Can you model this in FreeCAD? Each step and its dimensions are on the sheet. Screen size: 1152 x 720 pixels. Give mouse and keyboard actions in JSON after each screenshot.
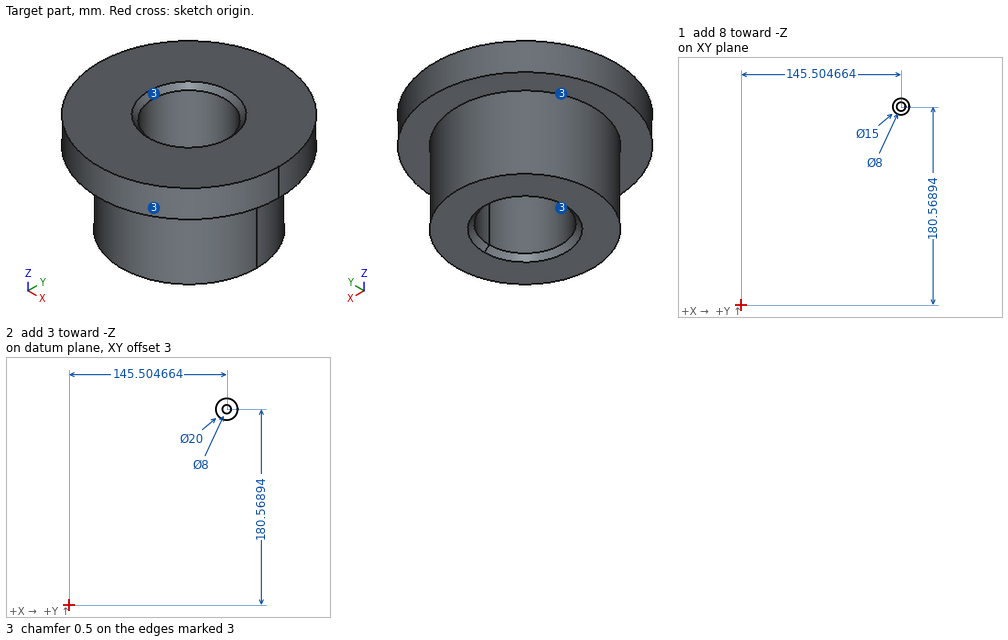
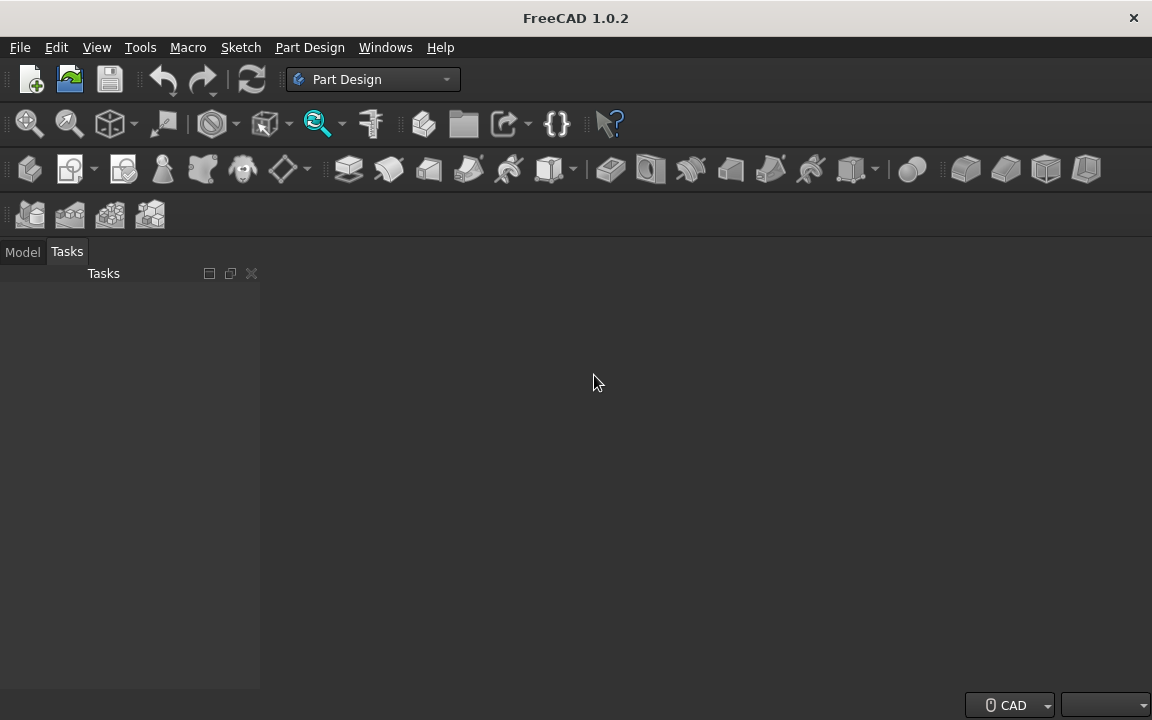
{"action": "left_click", "coordinate": [30, 80]}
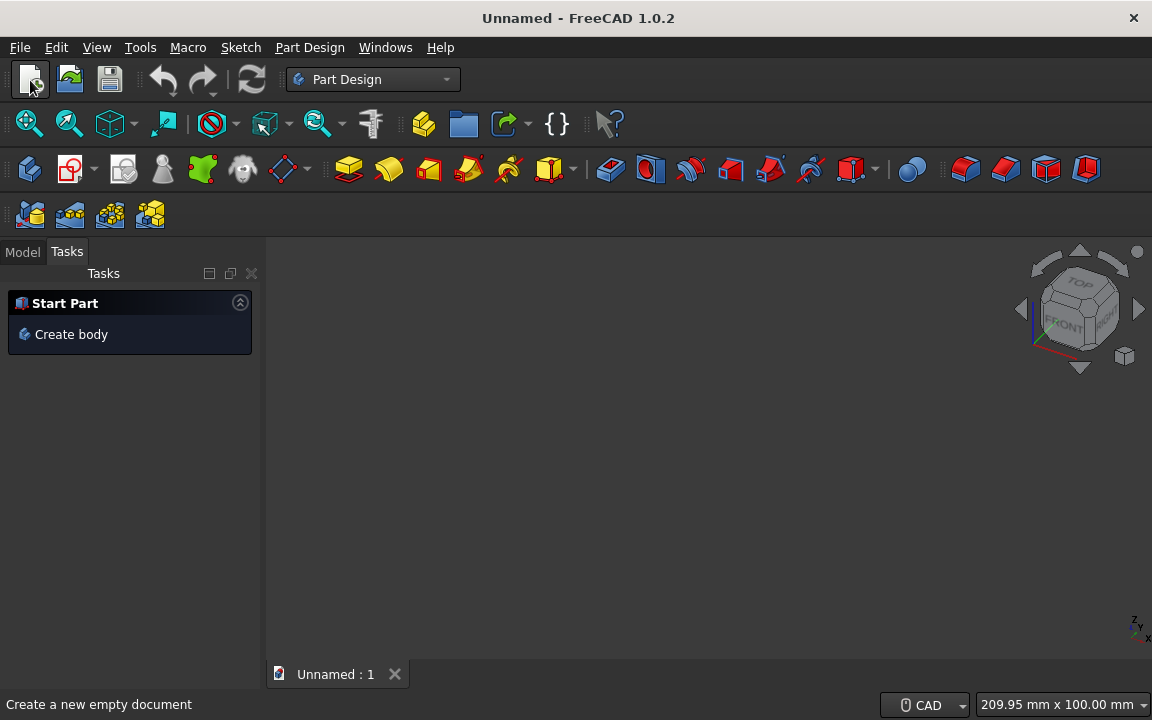
{"action": "left_click", "coordinate": [70, 170]}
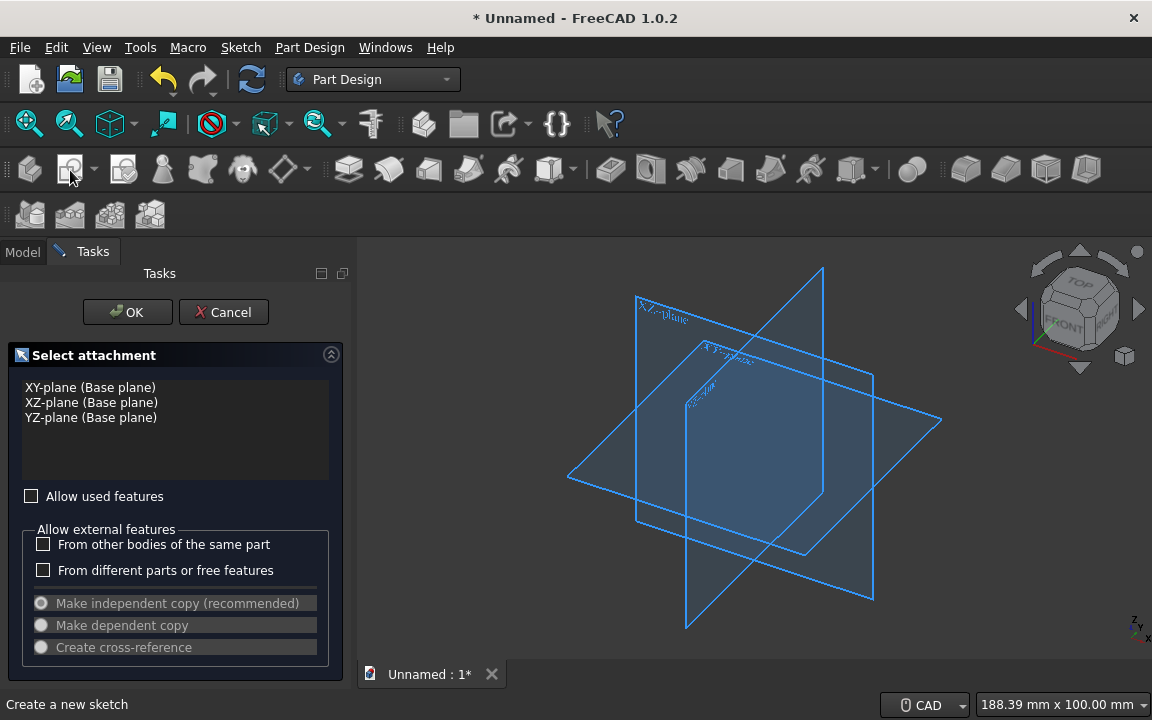
{"action": "left_click", "coordinate": [82, 388]}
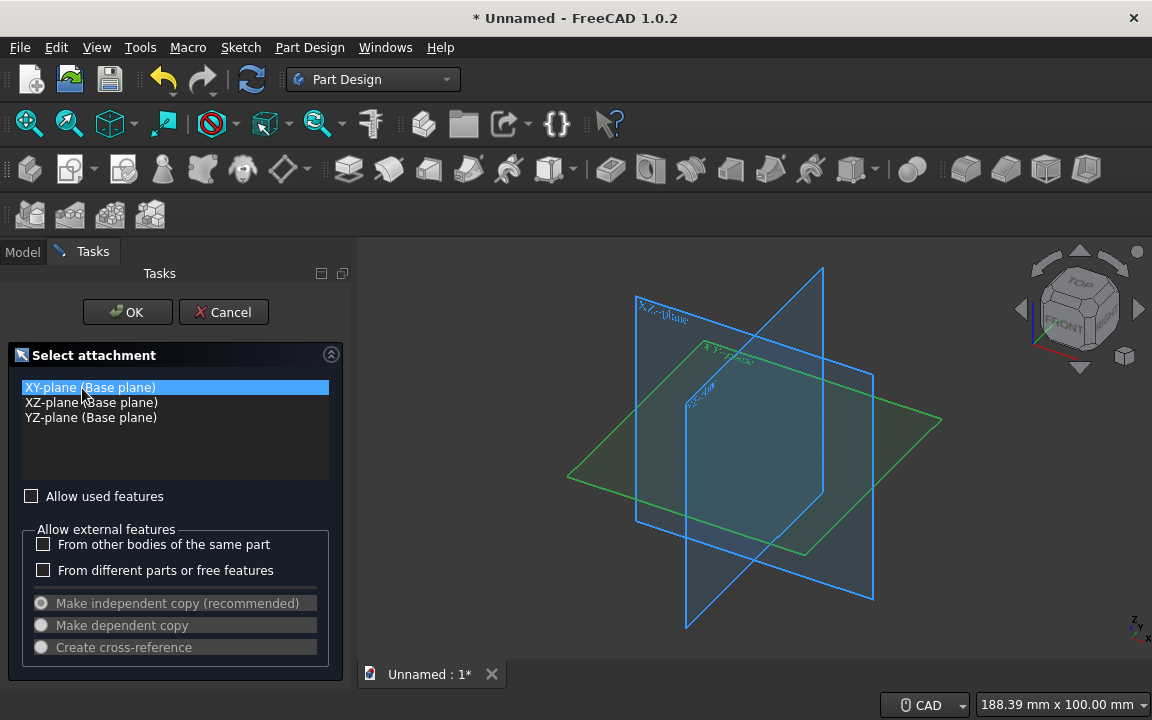
{"action": "left_click", "coordinate": [128, 312]}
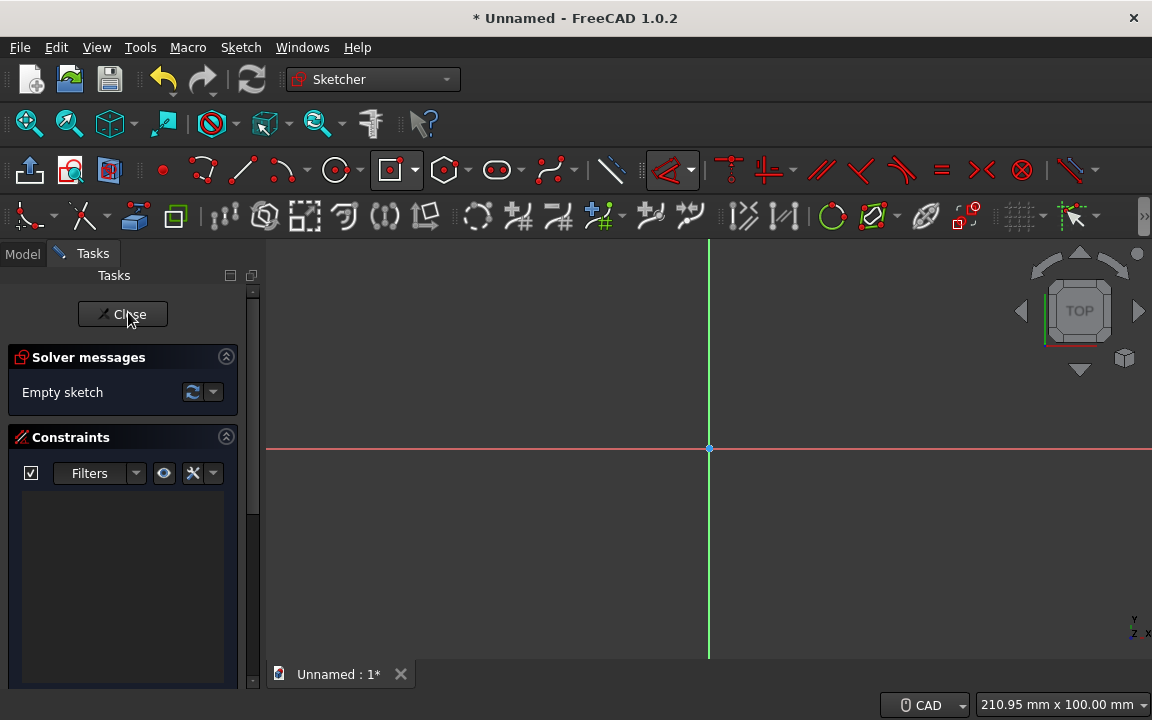
{"action": "scroll", "coordinate": [640, 449], "scroll_direction": "down", "scroll_amount": 5}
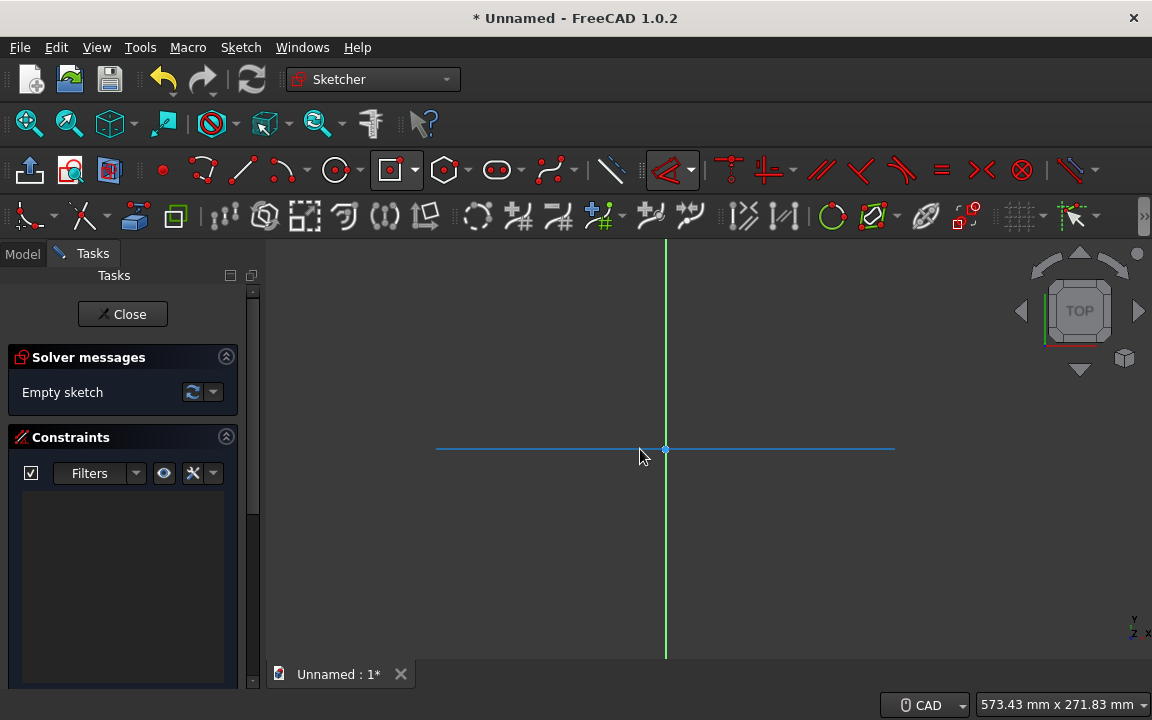
{"action": "scroll", "coordinate": [640, 449], "scroll_direction": "down", "scroll_amount": 5}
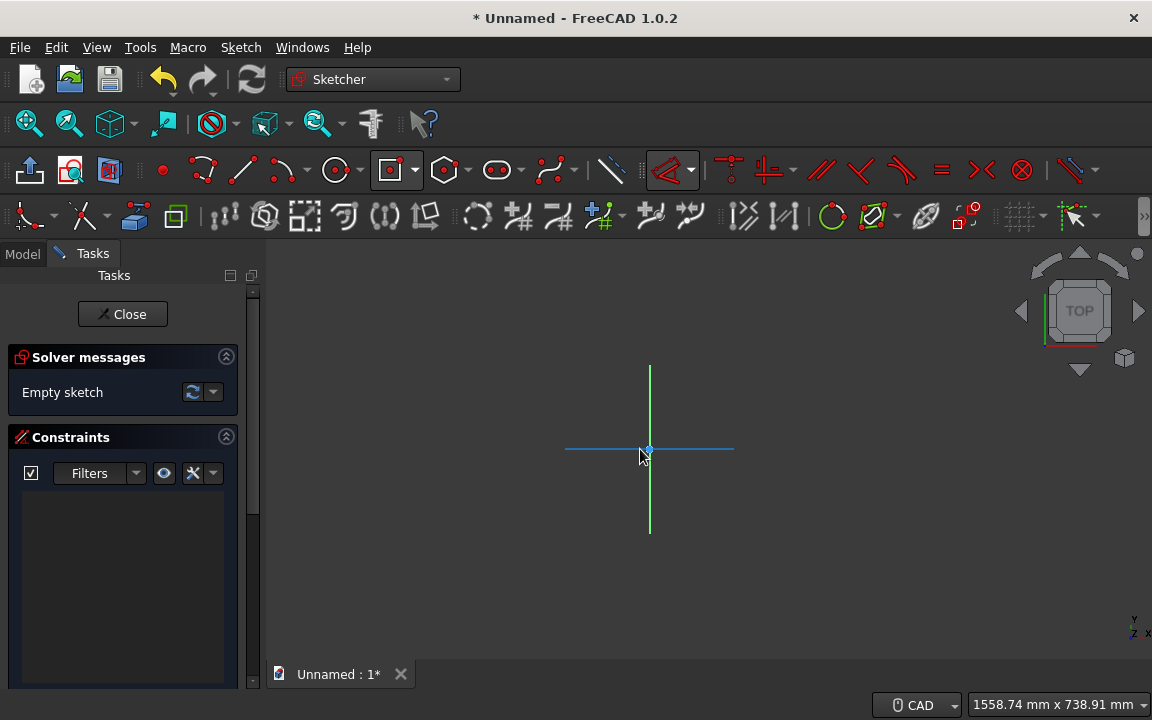
{"action": "scroll", "coordinate": [737, 341], "scroll_direction": "up", "scroll_amount": 15}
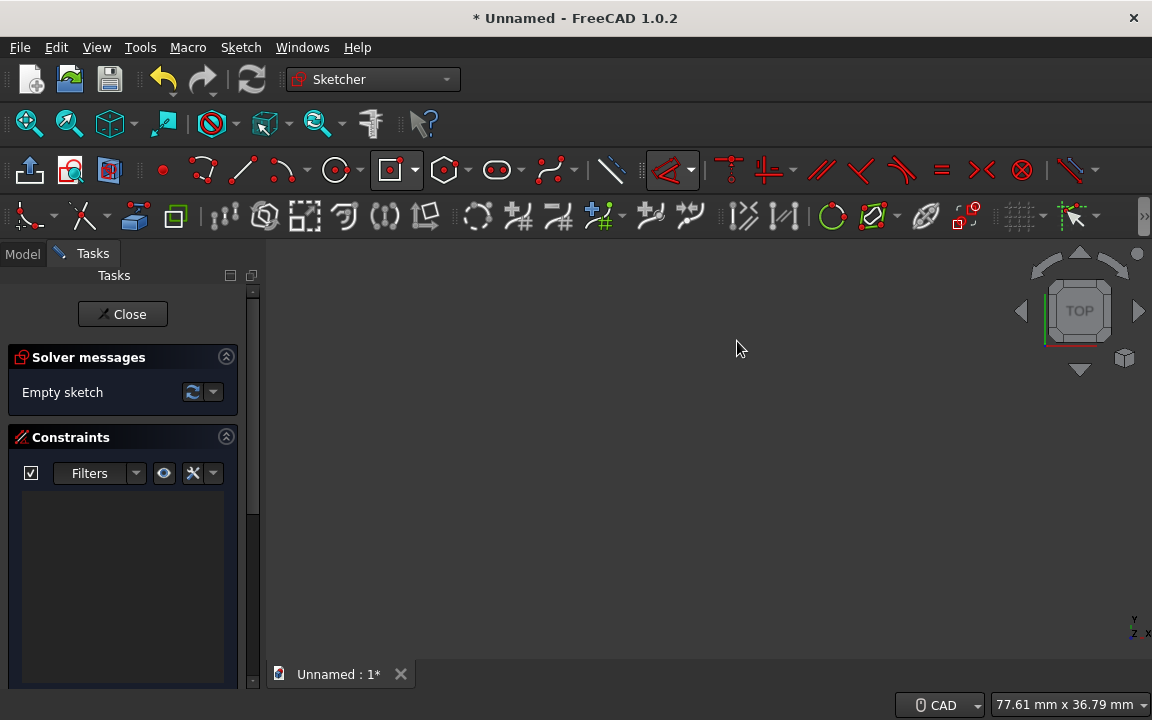
{"action": "scroll", "coordinate": [623, 460], "scroll_direction": "up", "scroll_amount": 2}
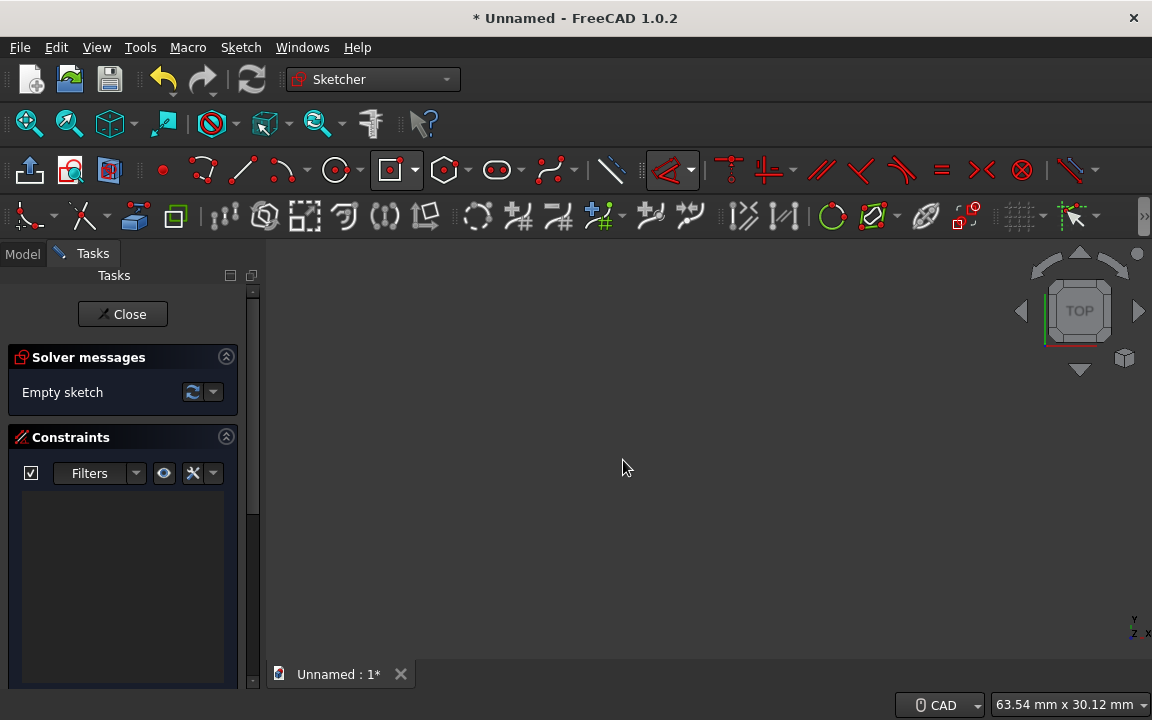
{"action": "key", "text": "g c"}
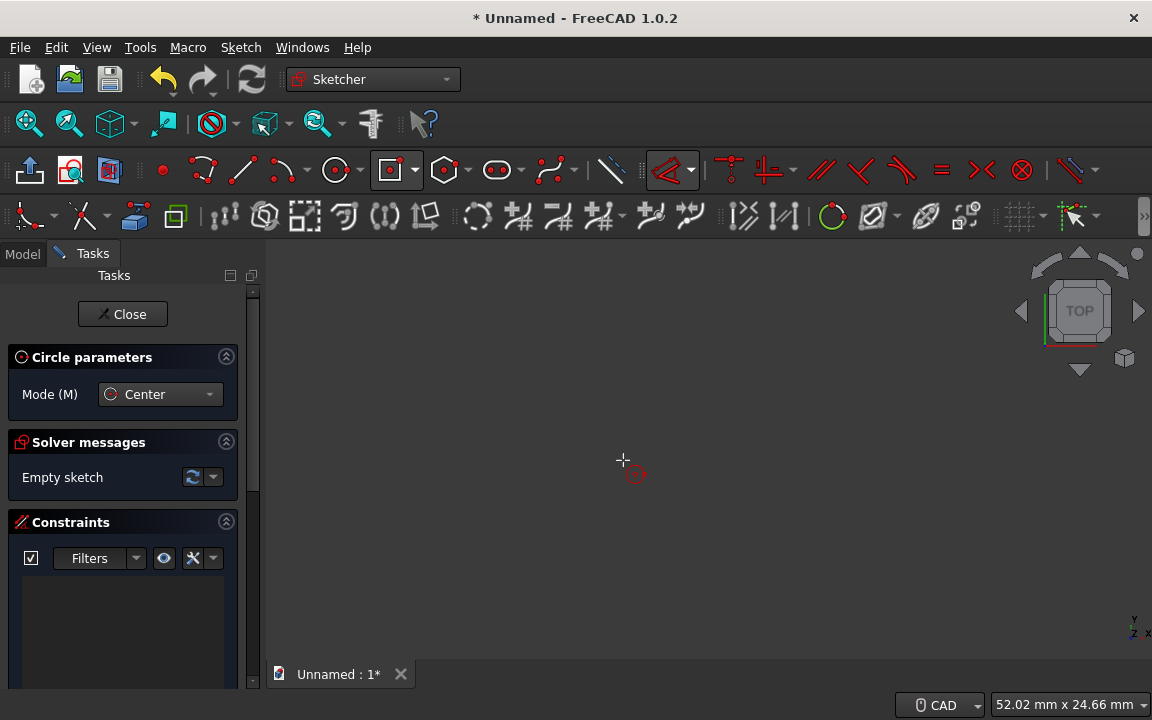
{"action": "left_click", "coordinate": [640, 449]}
{"action": "left_click", "coordinate": [730, 359]}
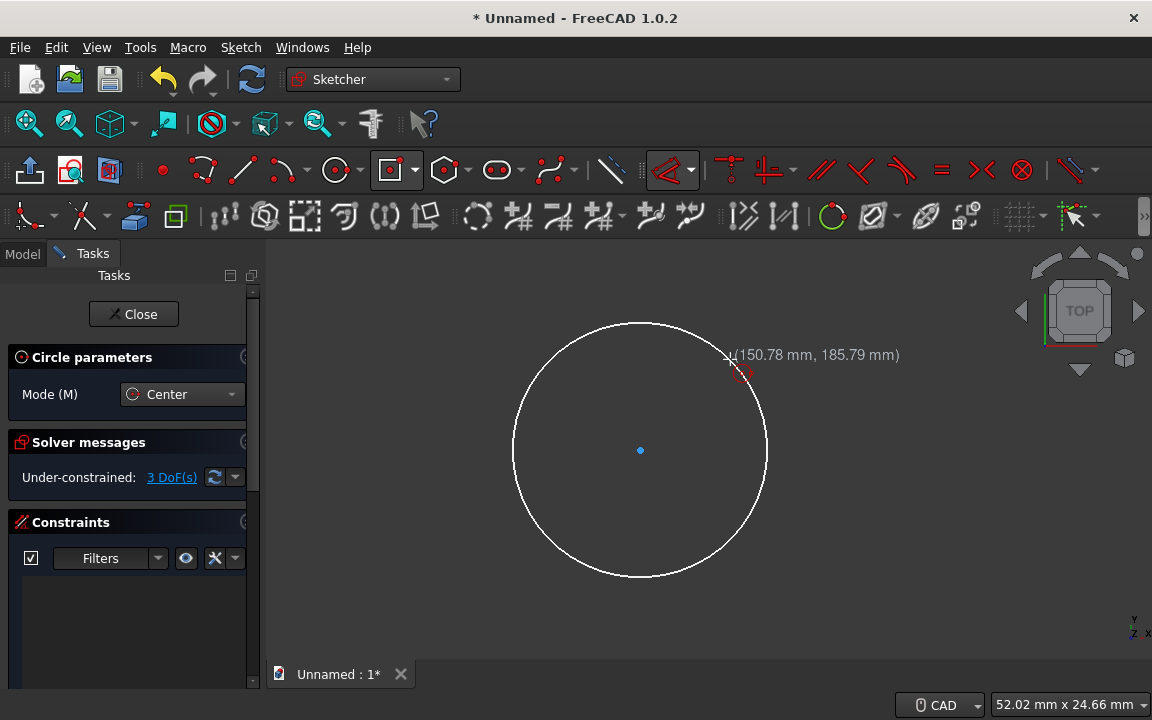
{"action": "left_click", "coordinate": [640, 450]}
{"action": "left_click", "coordinate": [688, 401]}
{"action": "key", "text": "Escape"}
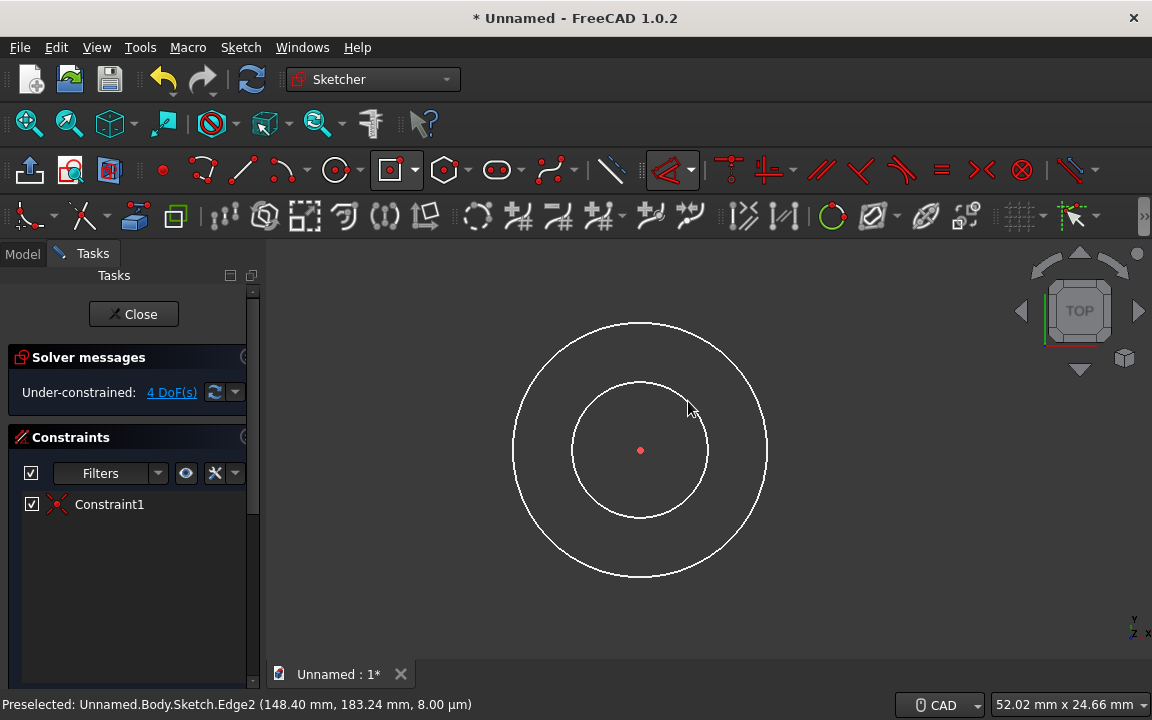
{"action": "key", "text": "d"}